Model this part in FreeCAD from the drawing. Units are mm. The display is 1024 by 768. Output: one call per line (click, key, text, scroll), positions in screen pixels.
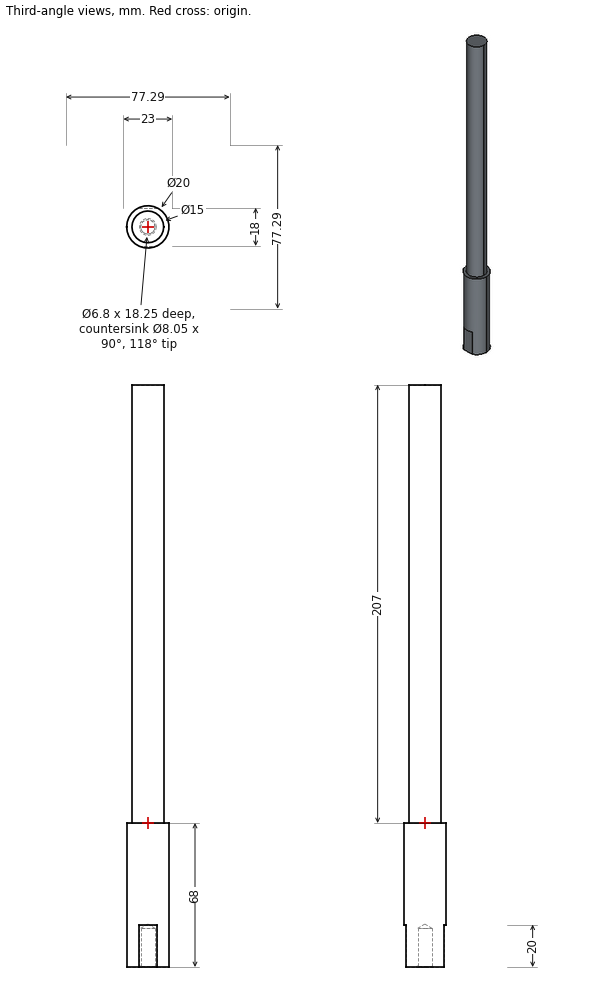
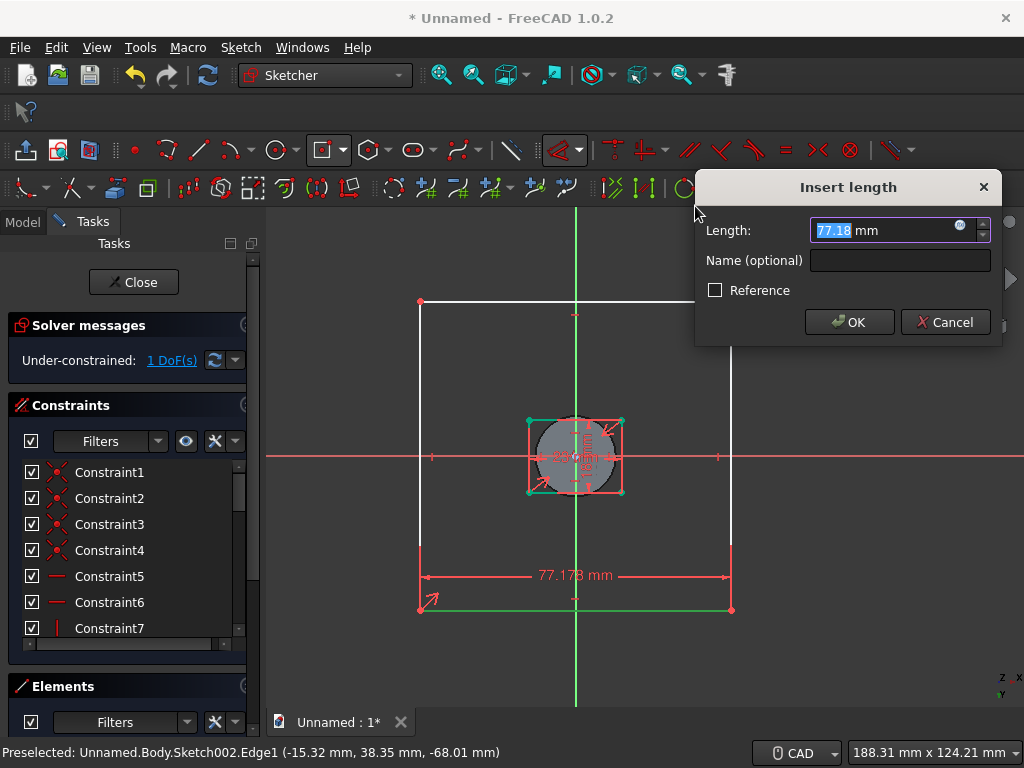
text(77.29)
key(Return)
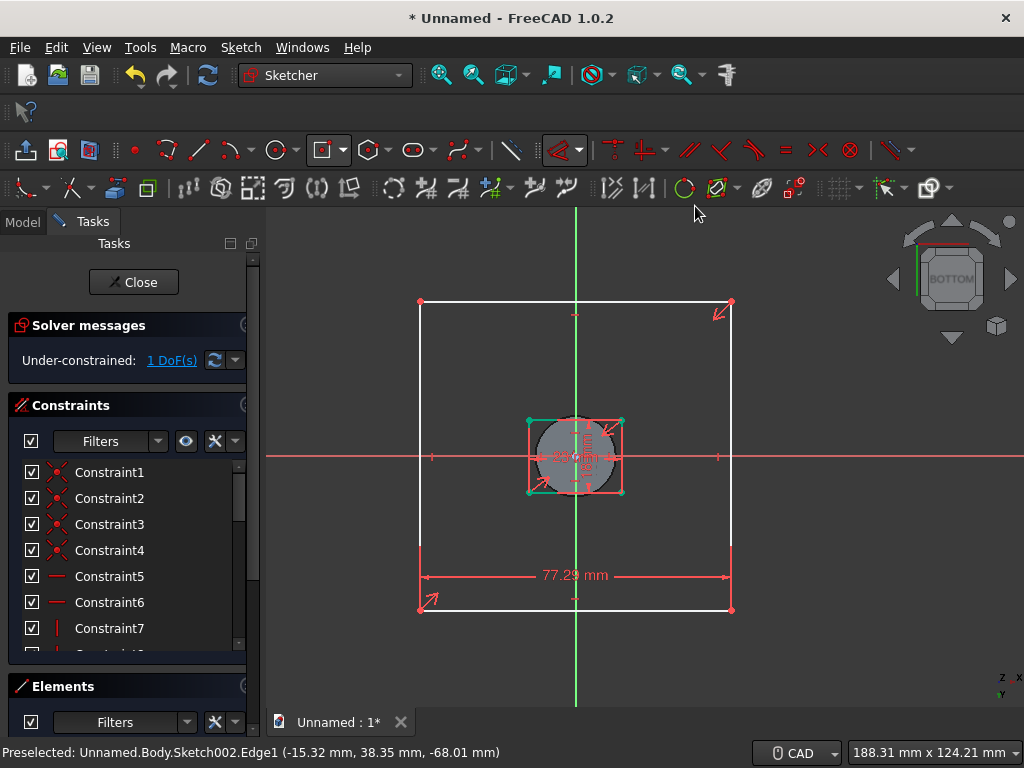
click(731, 518)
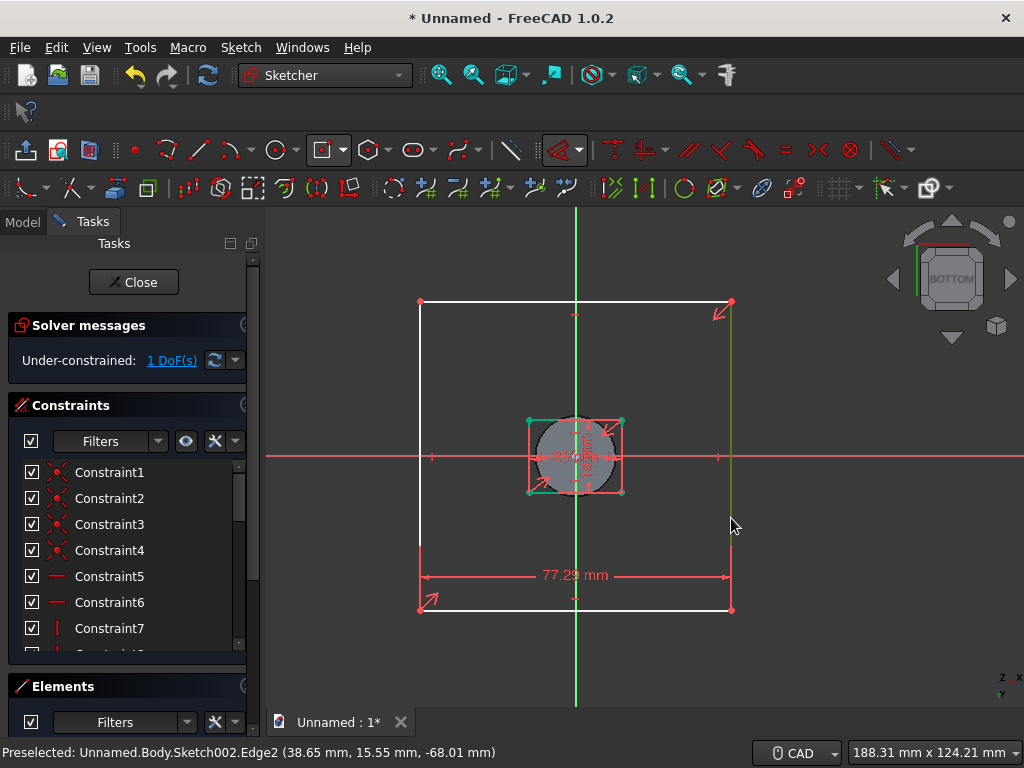
click(582, 150)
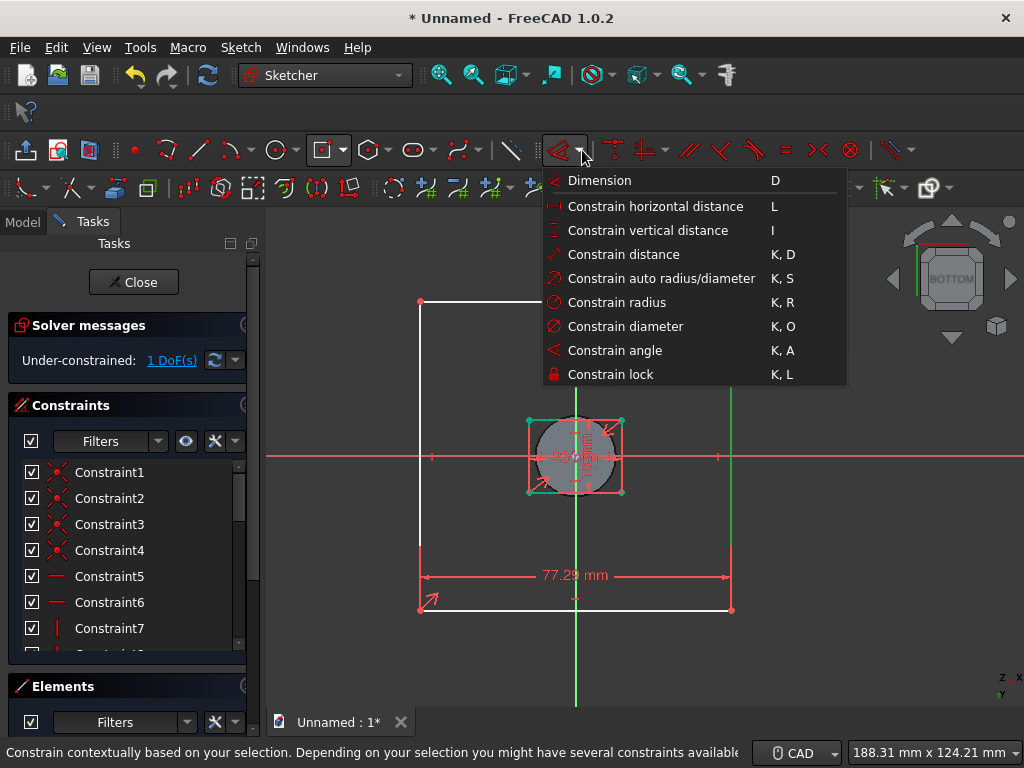
click(695, 230)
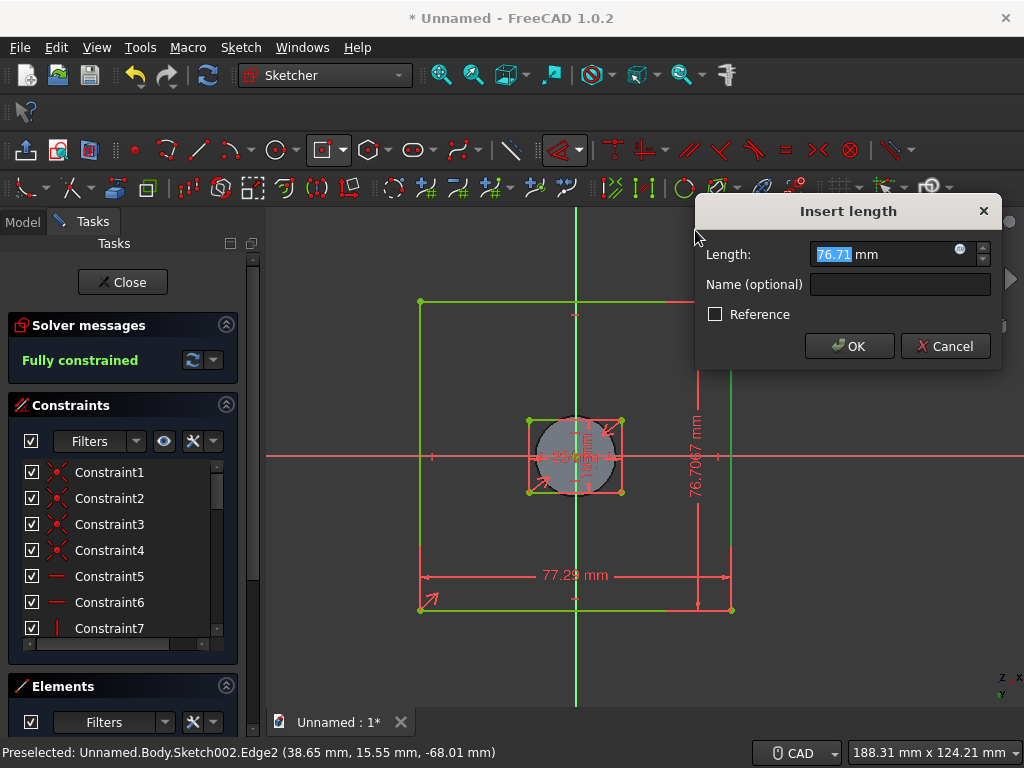
text(77.29)
key(Return)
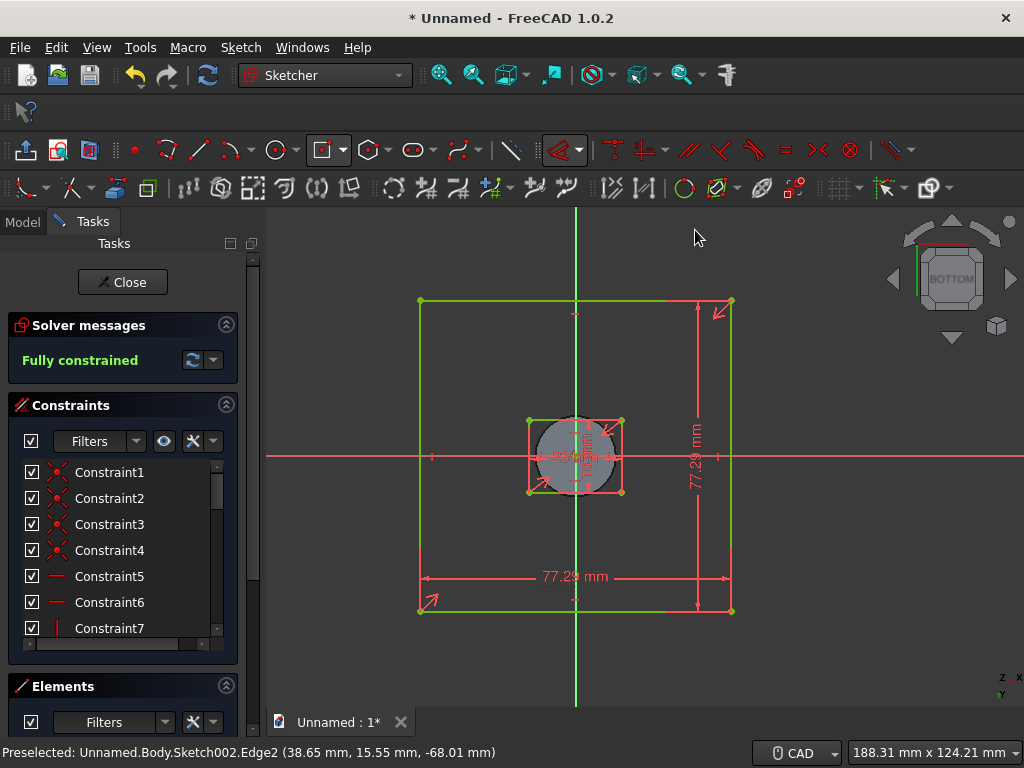
click(123, 282)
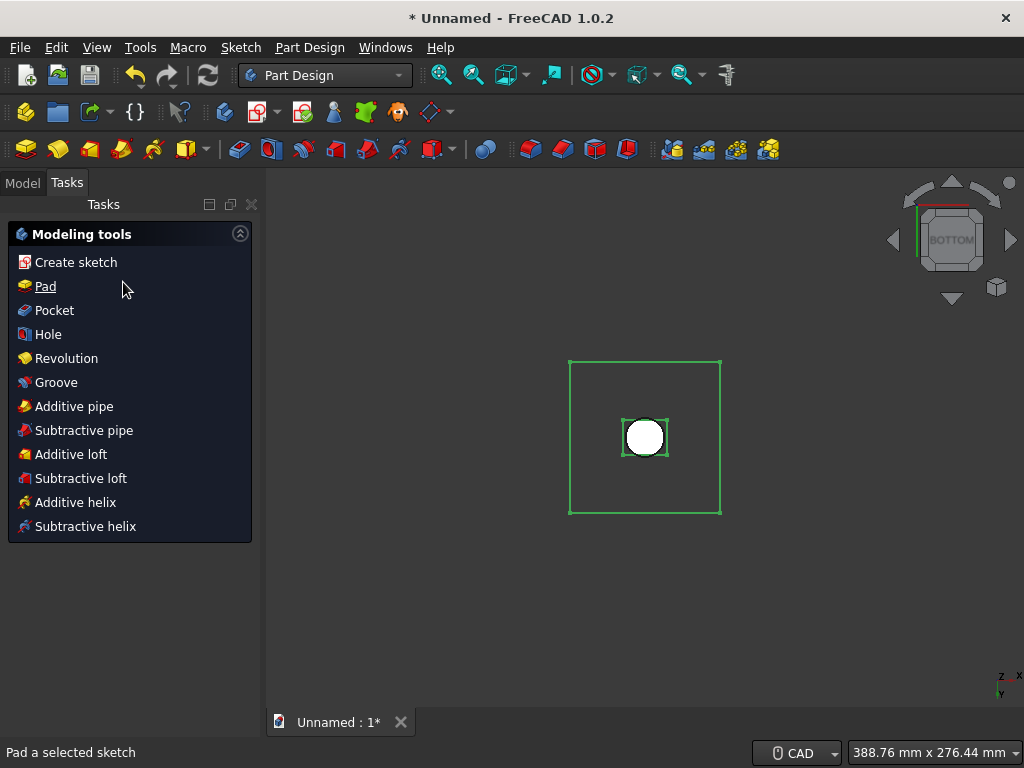
click(240, 150)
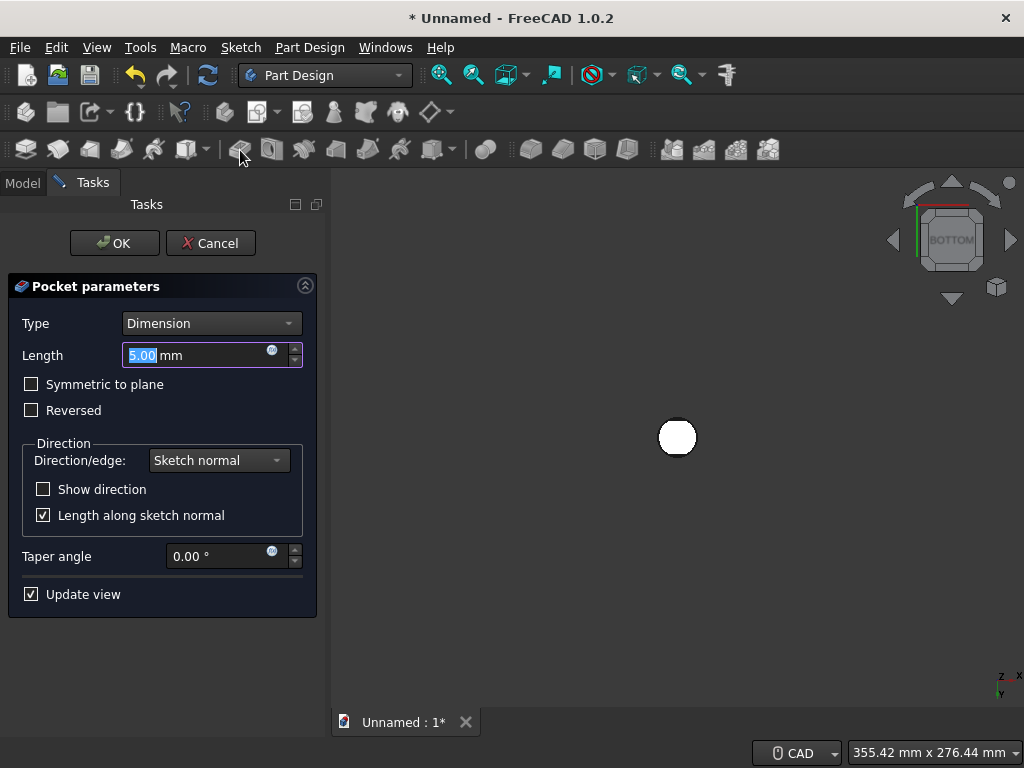
text(20)
key(Tab)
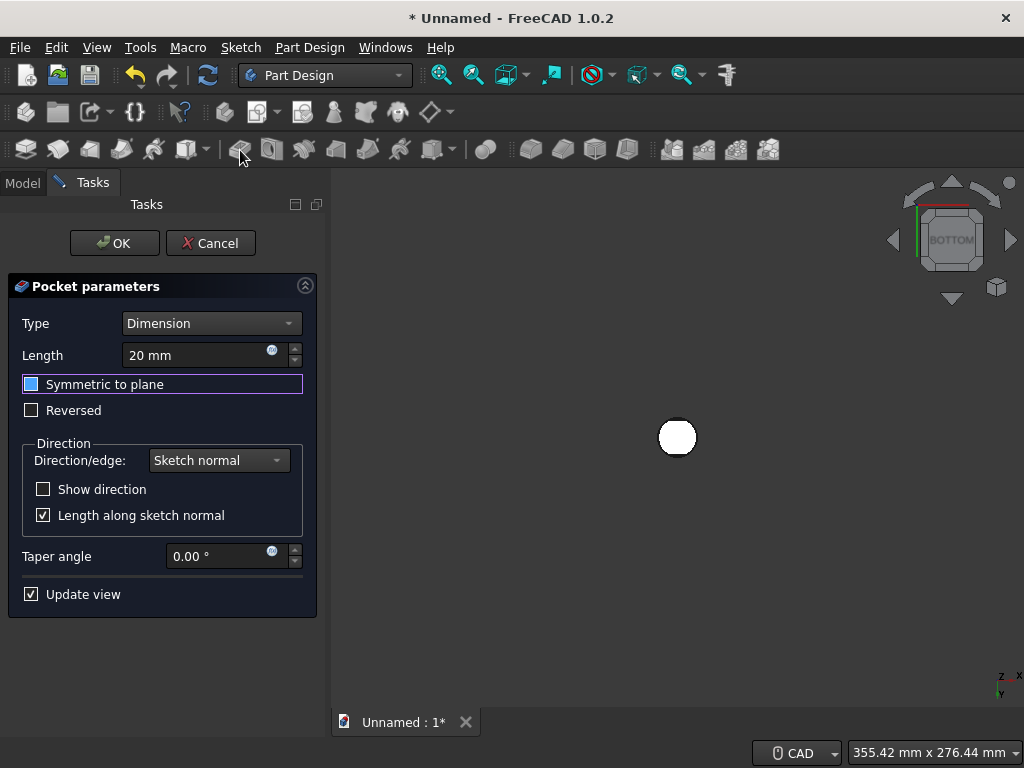
click(115, 243)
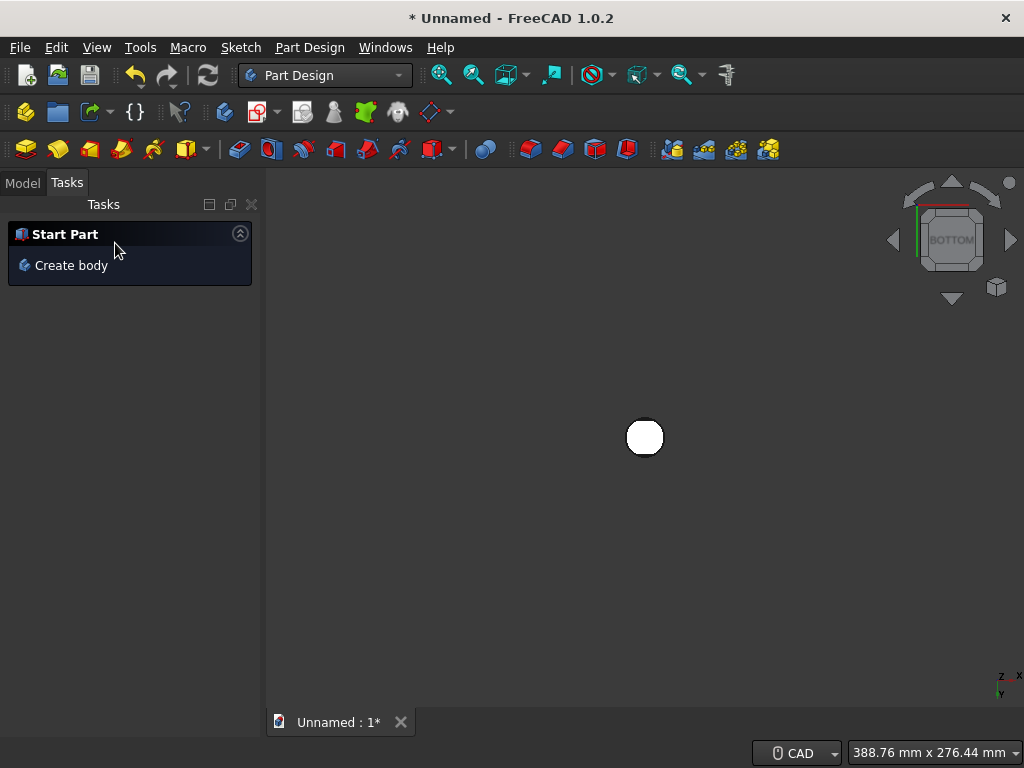
click(442, 76)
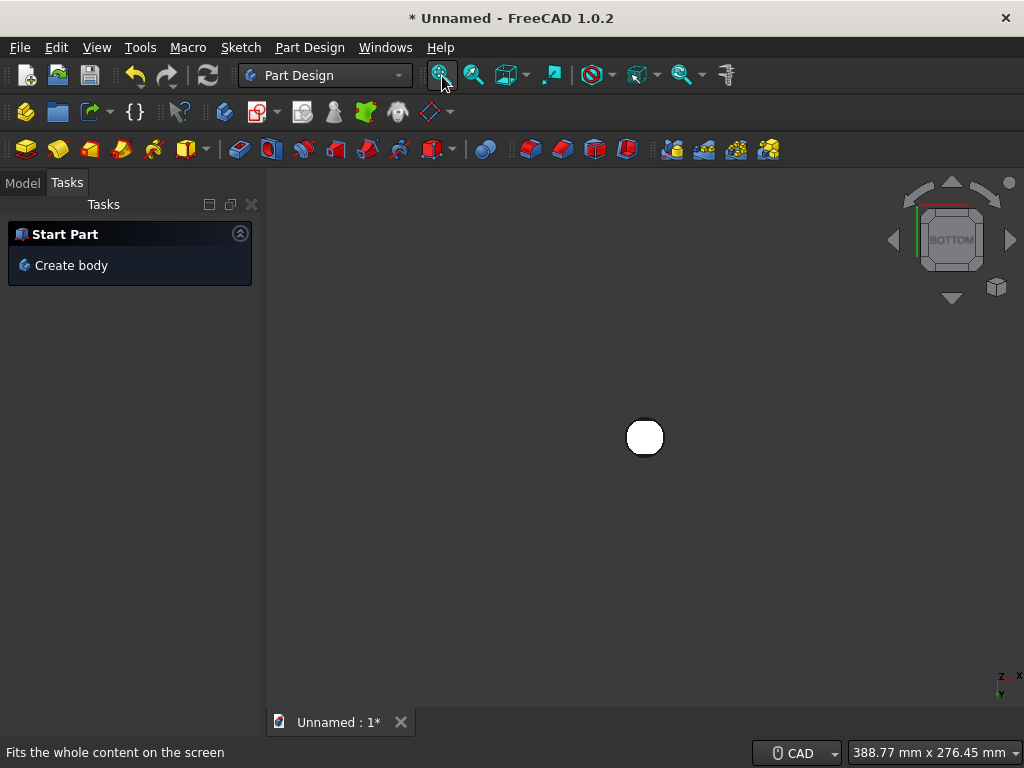
click(645, 436)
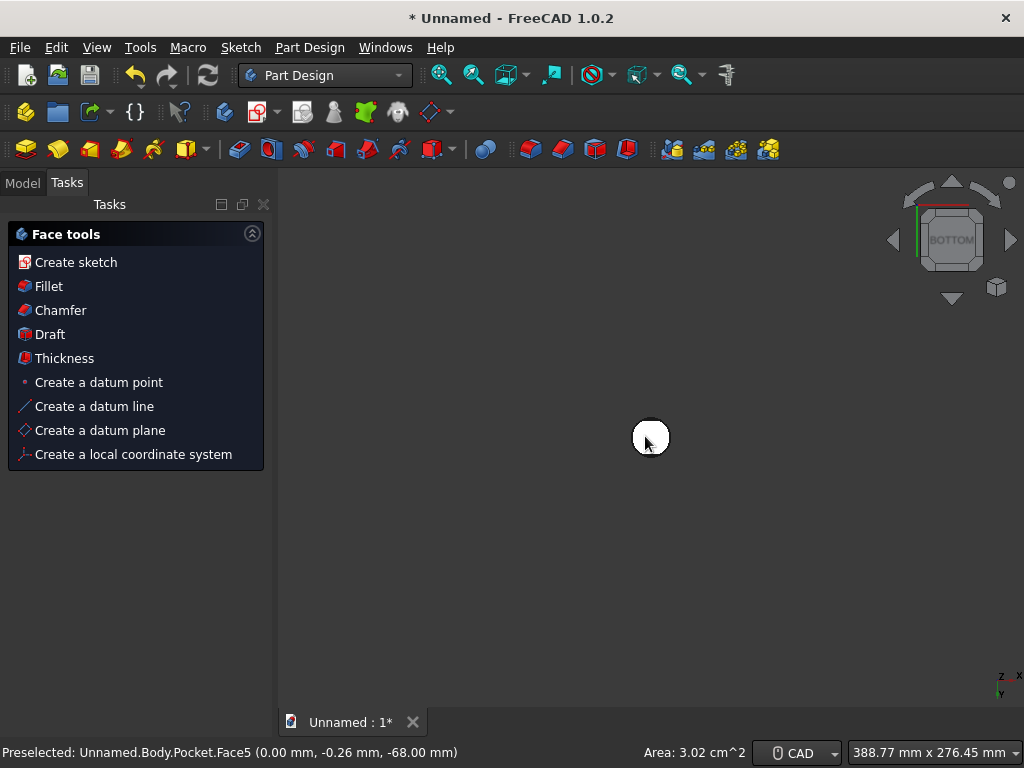
click(258, 112)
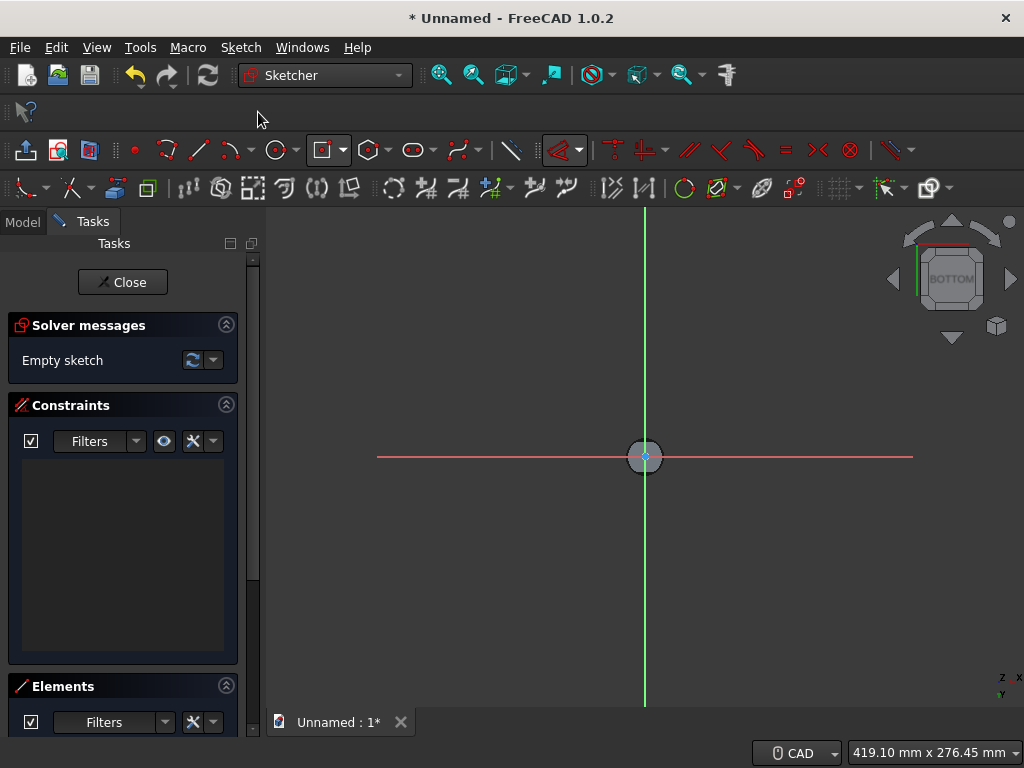
scroll(649, 457, up, 15)